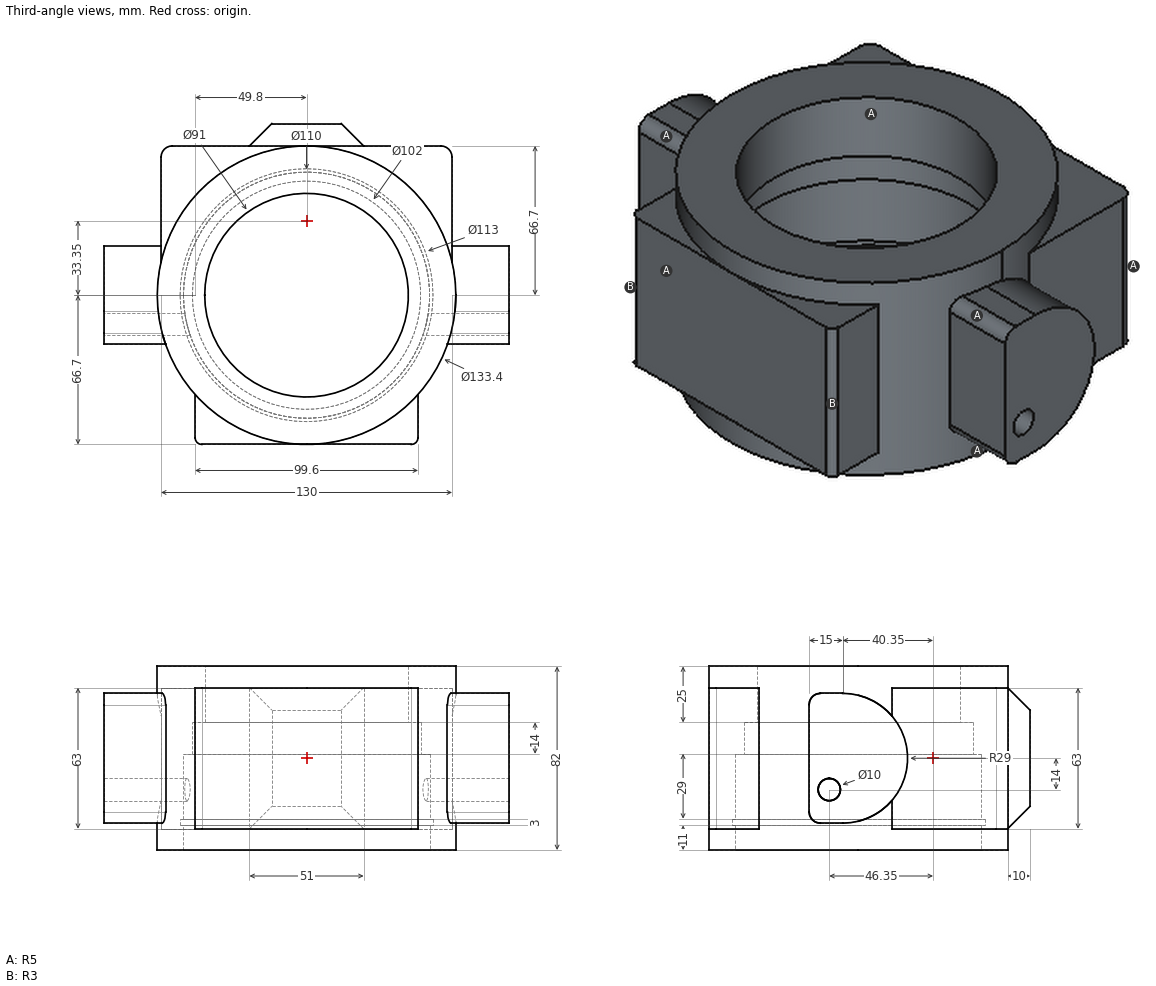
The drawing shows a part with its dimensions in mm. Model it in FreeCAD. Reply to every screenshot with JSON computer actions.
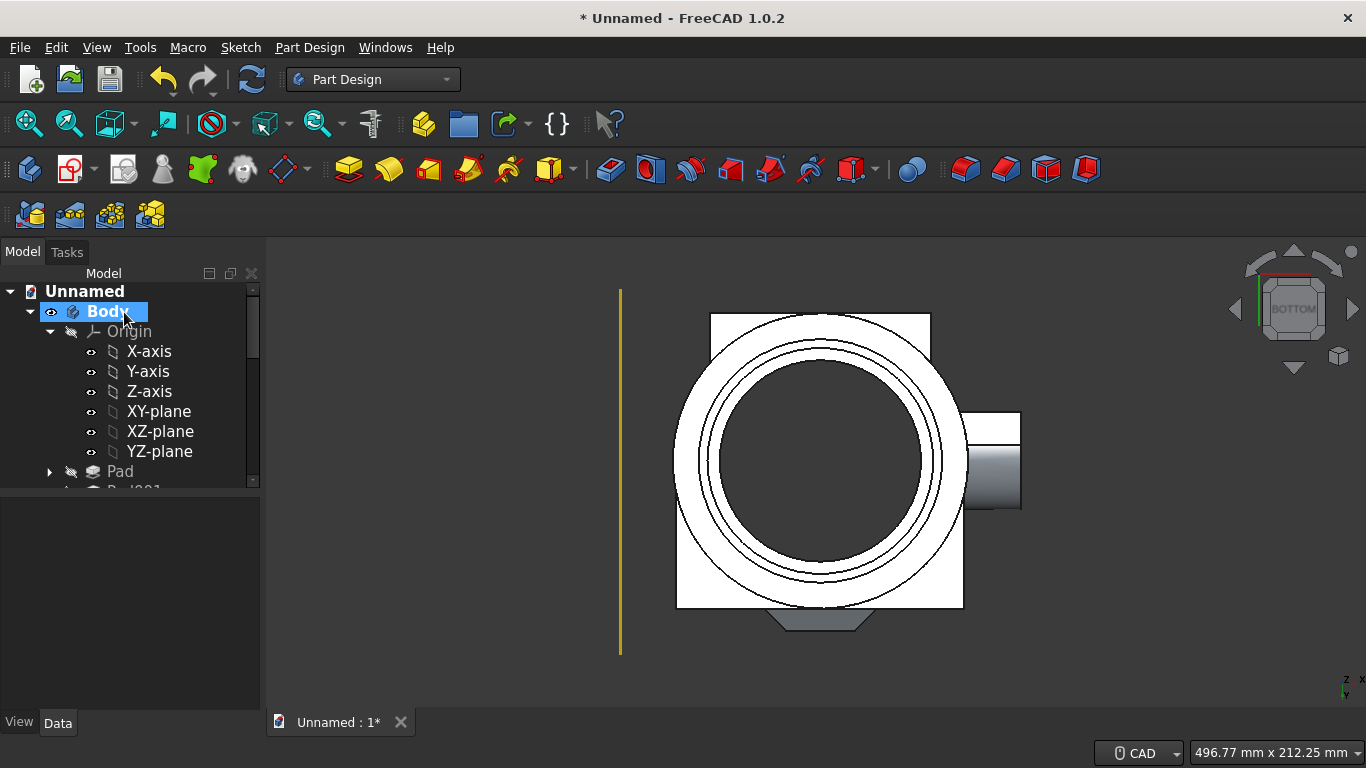
{"action": "scroll", "coordinate": [100, 387], "scroll_direction": "down", "scroll_amount": 3}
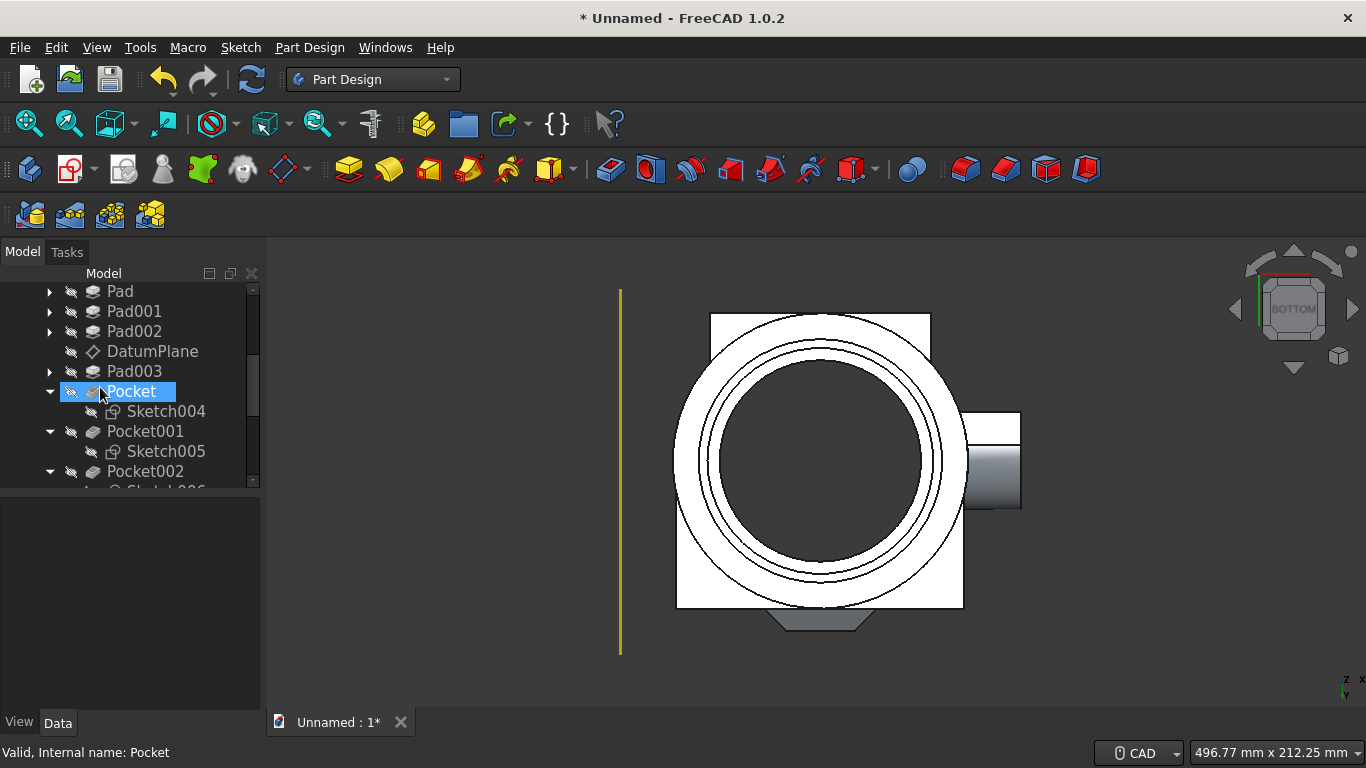
{"action": "scroll", "coordinate": [140, 387], "scroll_direction": "up", "scroll_amount": 15}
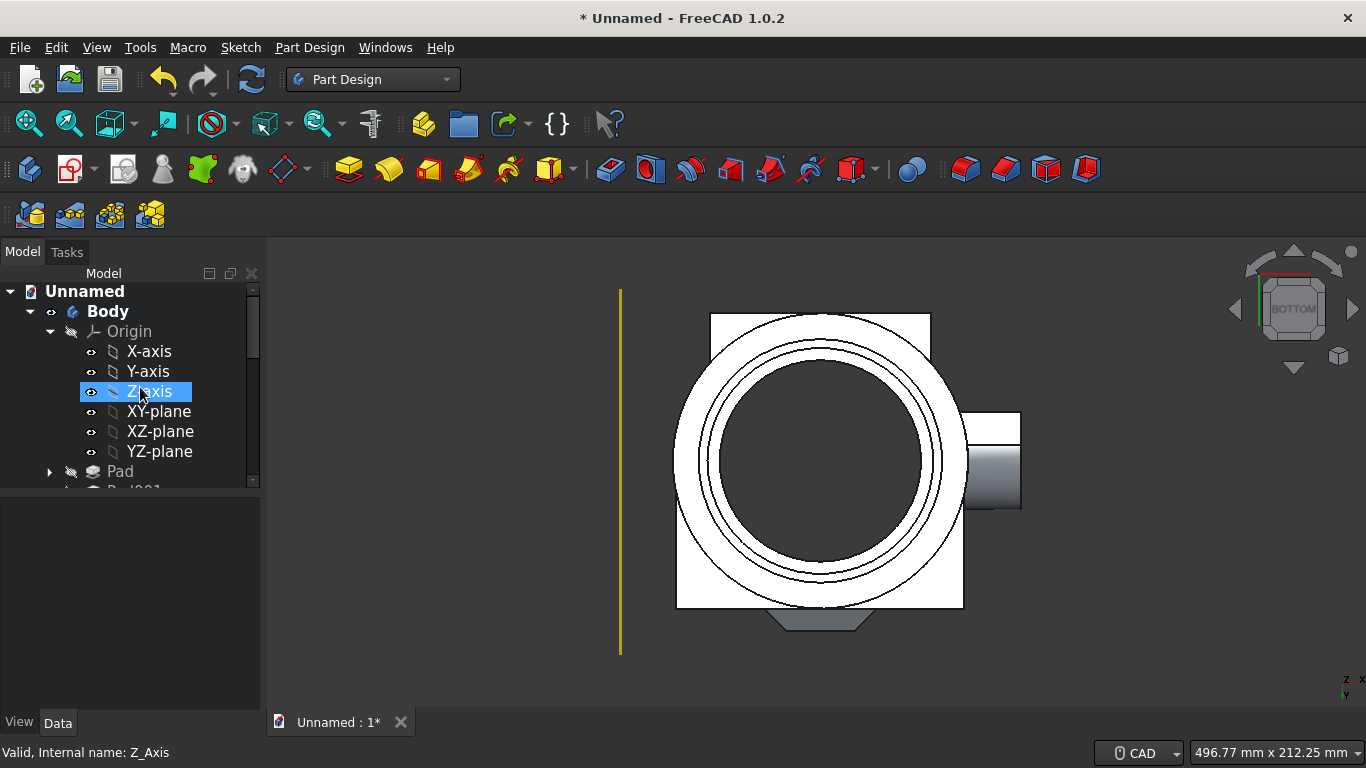
{"action": "scroll", "coordinate": [100, 387], "scroll_direction": "down", "scroll_amount": 6}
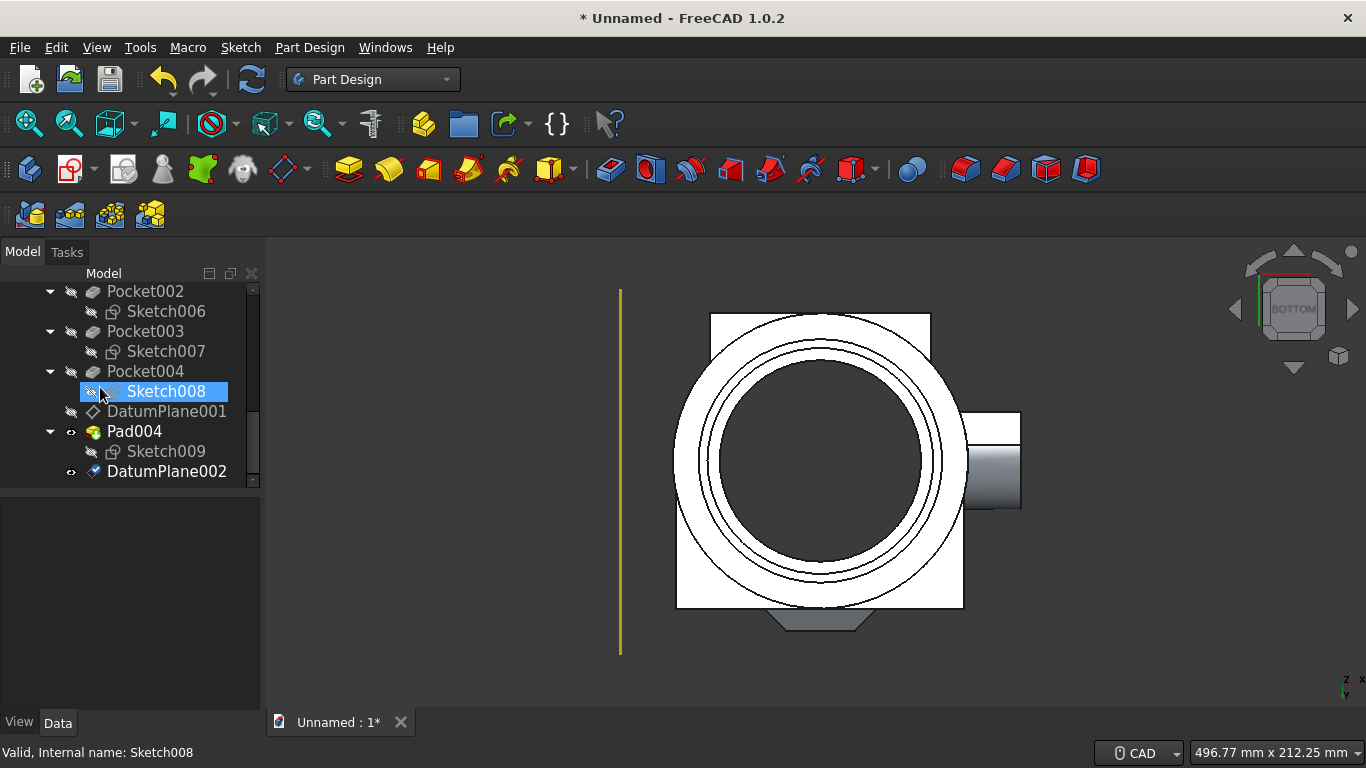
{"action": "left_click", "coordinate": [116, 472]}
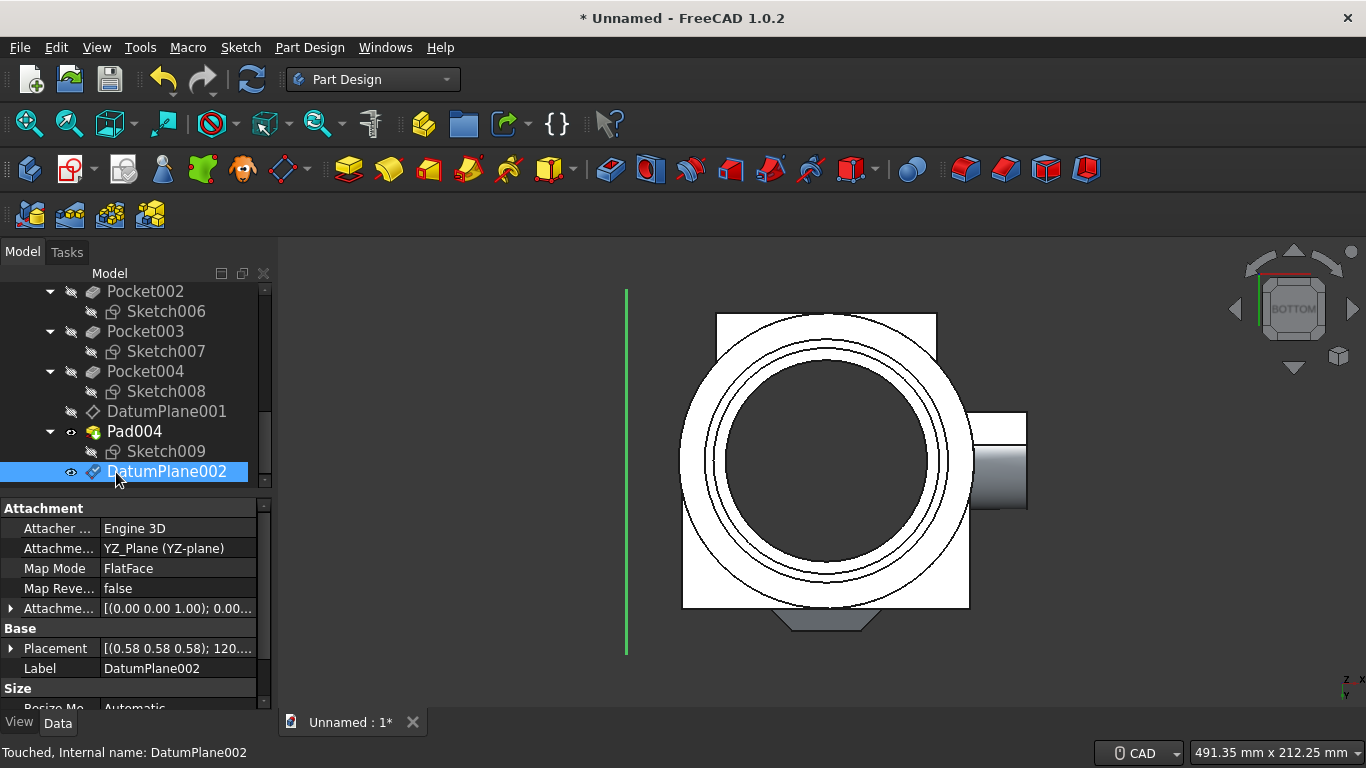
{"action": "left_click", "coordinate": [70, 170]}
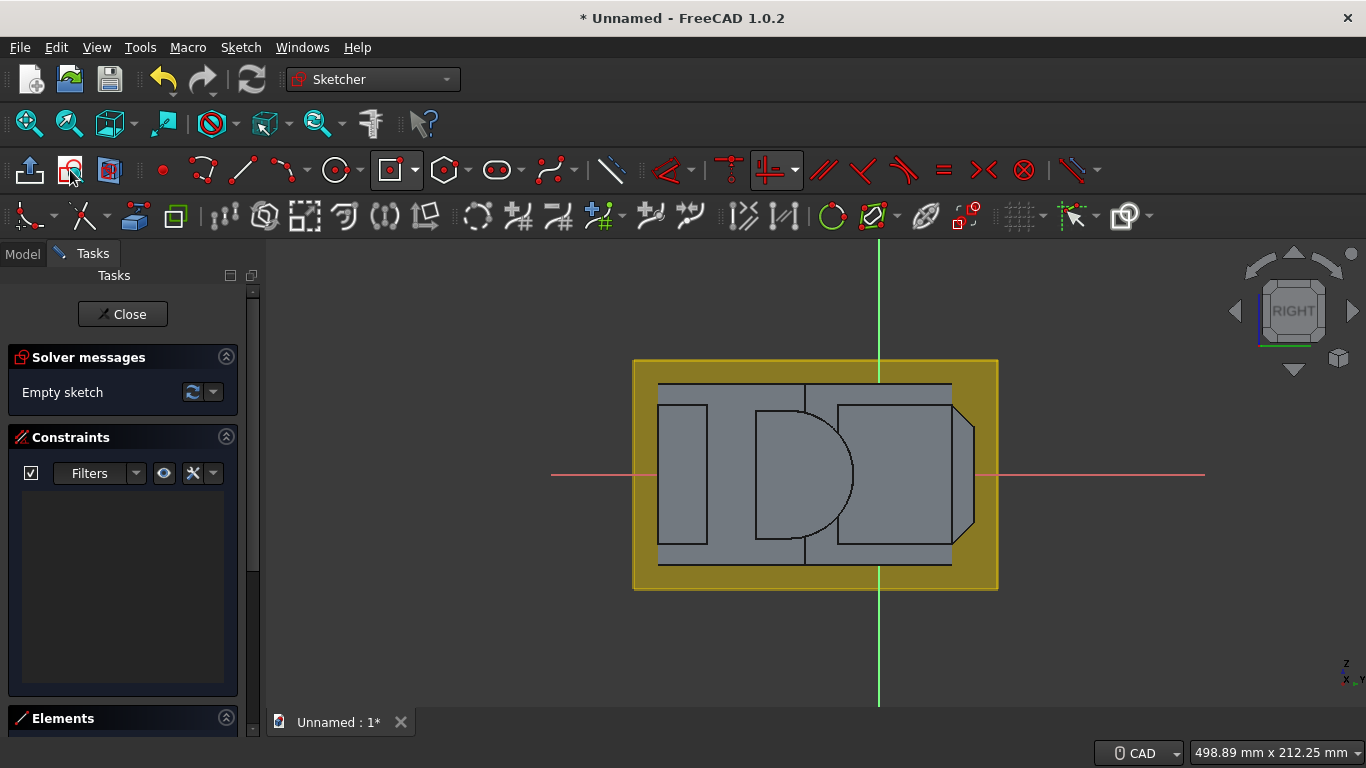
{"action": "key", "text": "q s"}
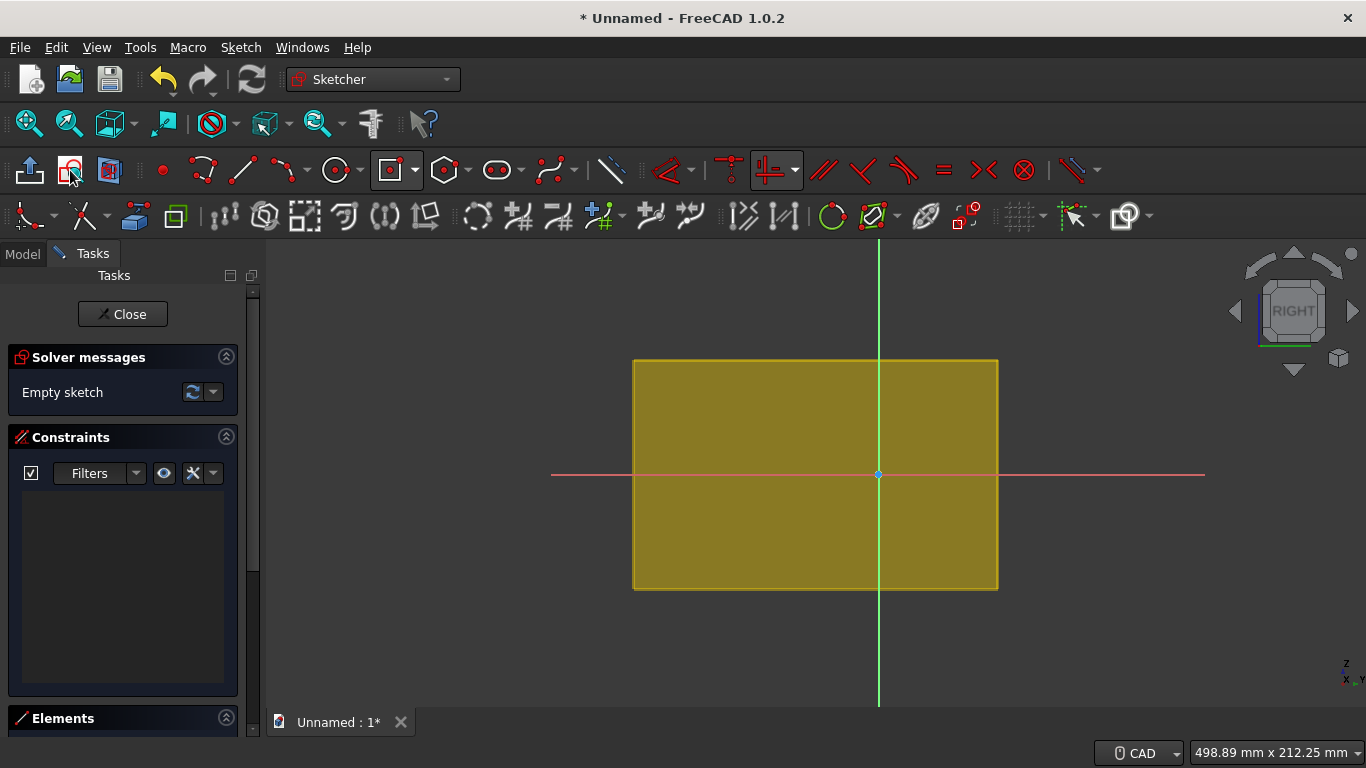
{"action": "scroll", "coordinate": [875, 476], "scroll_direction": "up", "scroll_amount": 4}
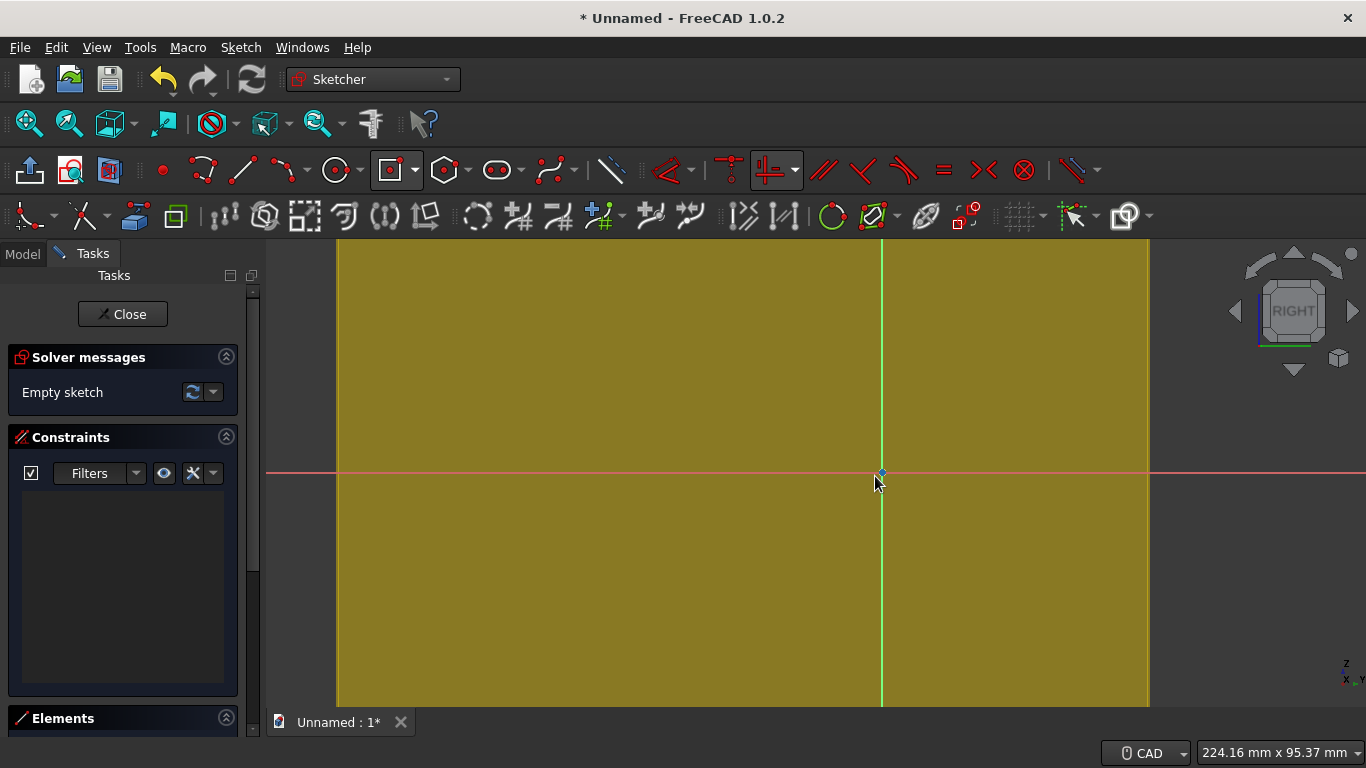
{"action": "key", "text": "g m"}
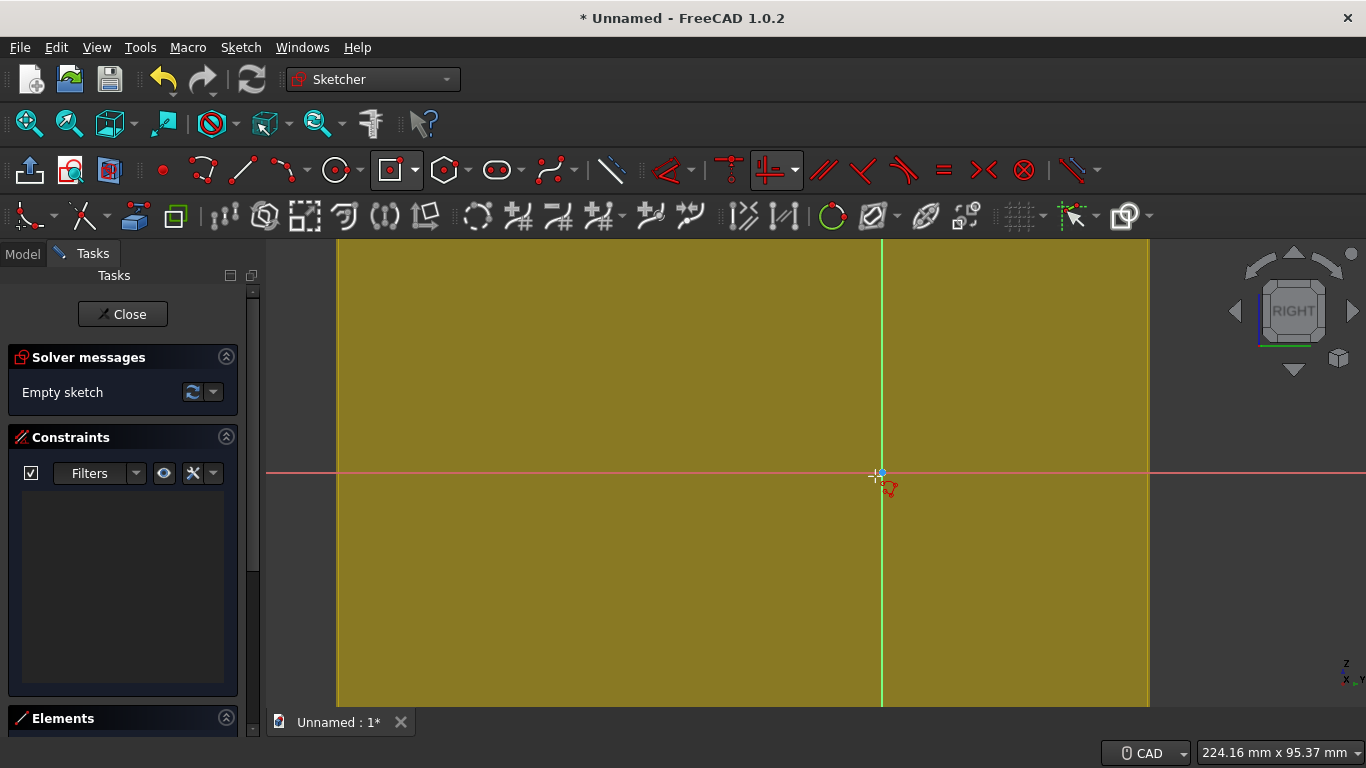
{"action": "left_click", "coordinate": [684, 330]}
{"action": "left_click", "coordinate": [611, 330]}
{"action": "left_click", "coordinate": [611, 615]}
{"action": "left_click", "coordinate": [684, 615]}
{"action": "right_click", "coordinate": [684, 615]}